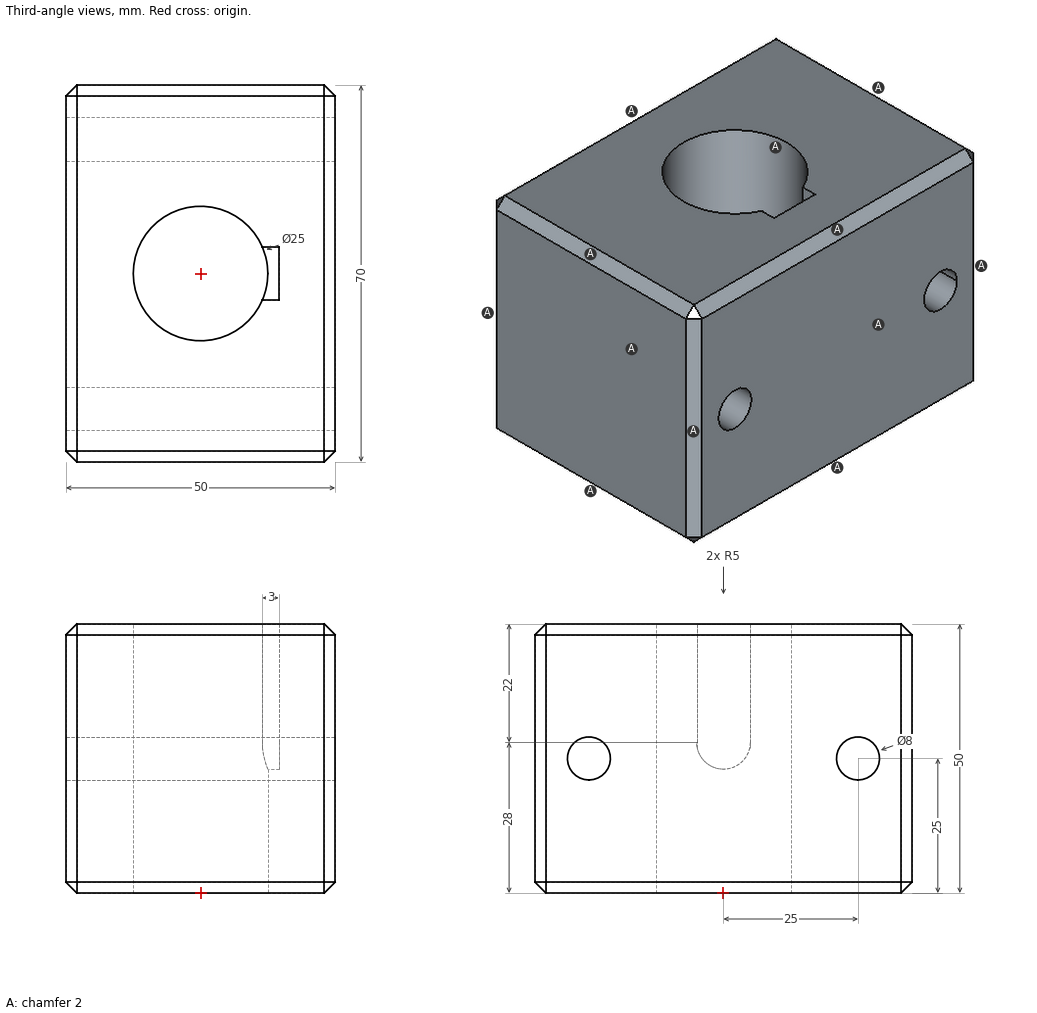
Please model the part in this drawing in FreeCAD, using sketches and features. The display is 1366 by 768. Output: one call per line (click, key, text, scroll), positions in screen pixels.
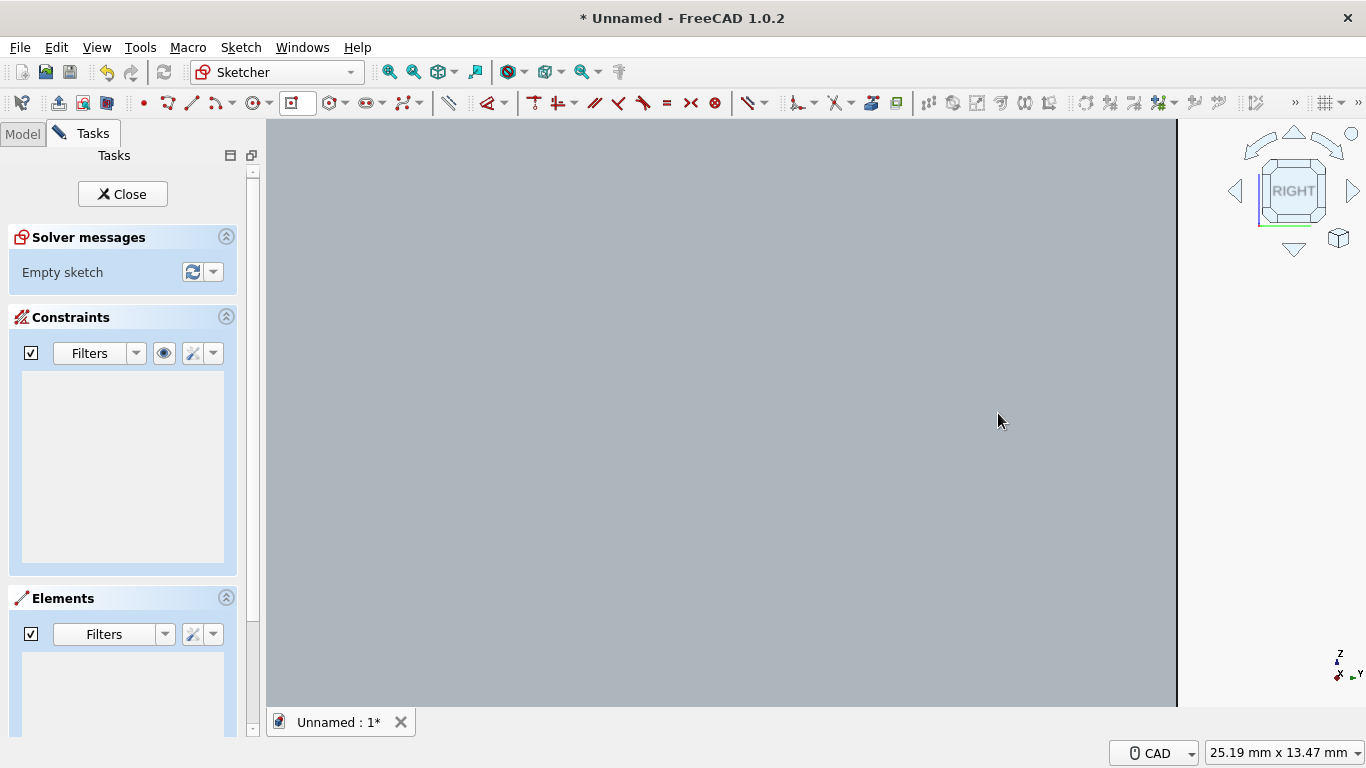
click(254, 104)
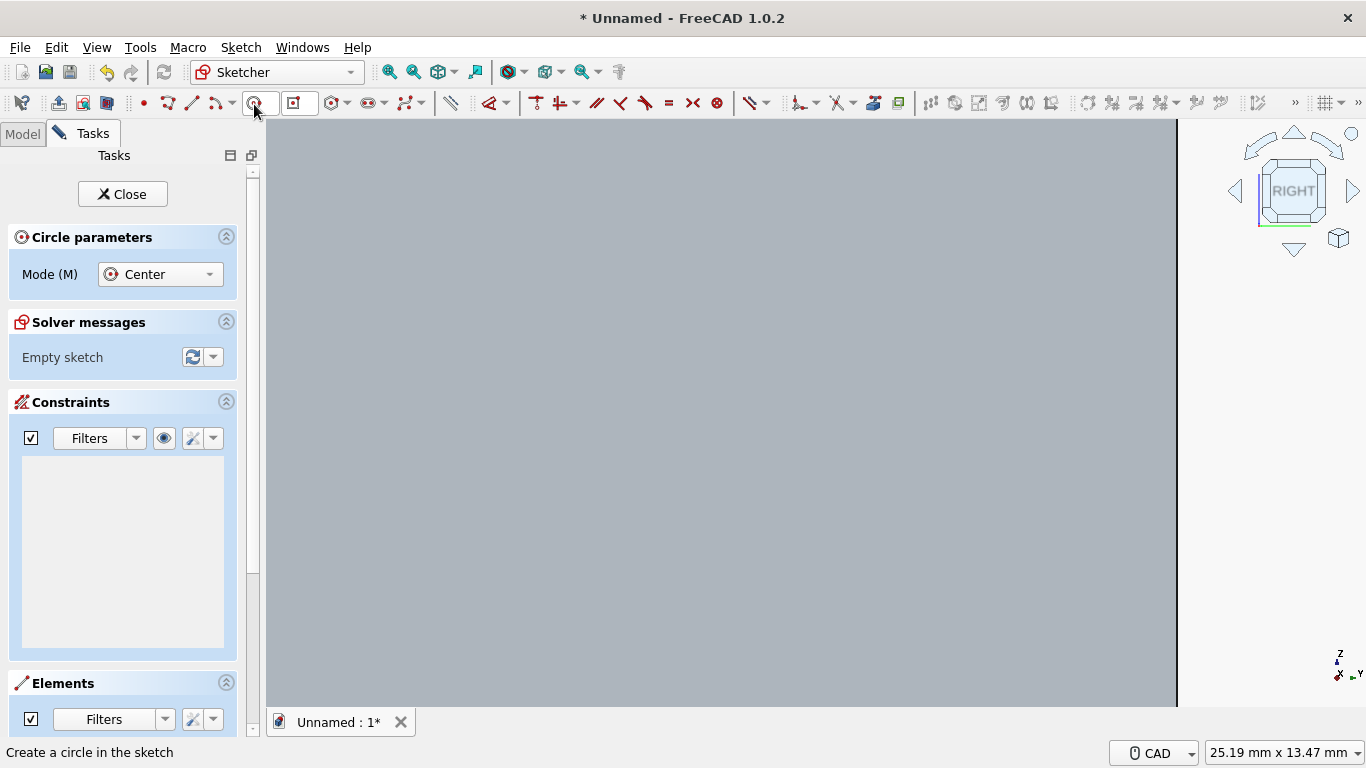
click(741, 410)
move(864, 286)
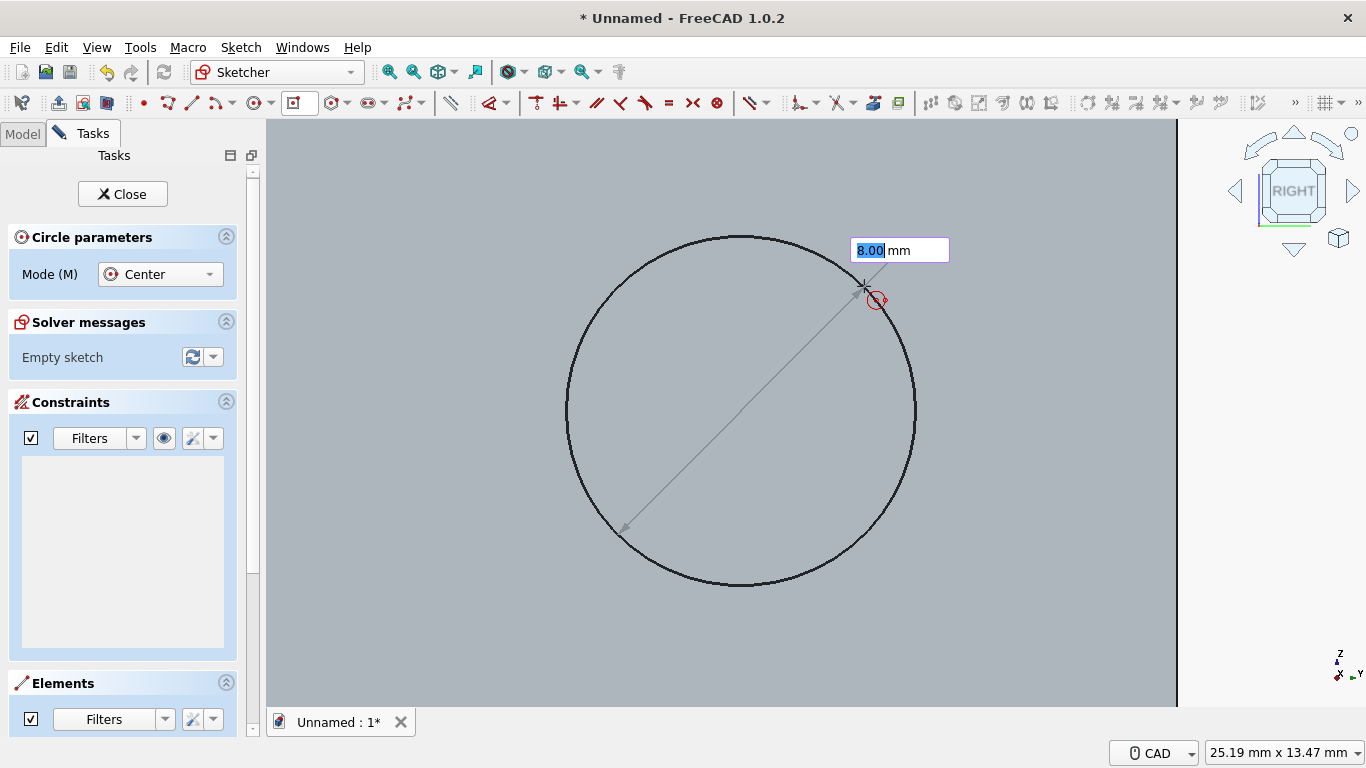
text(8)
key(Return)
key(Escape)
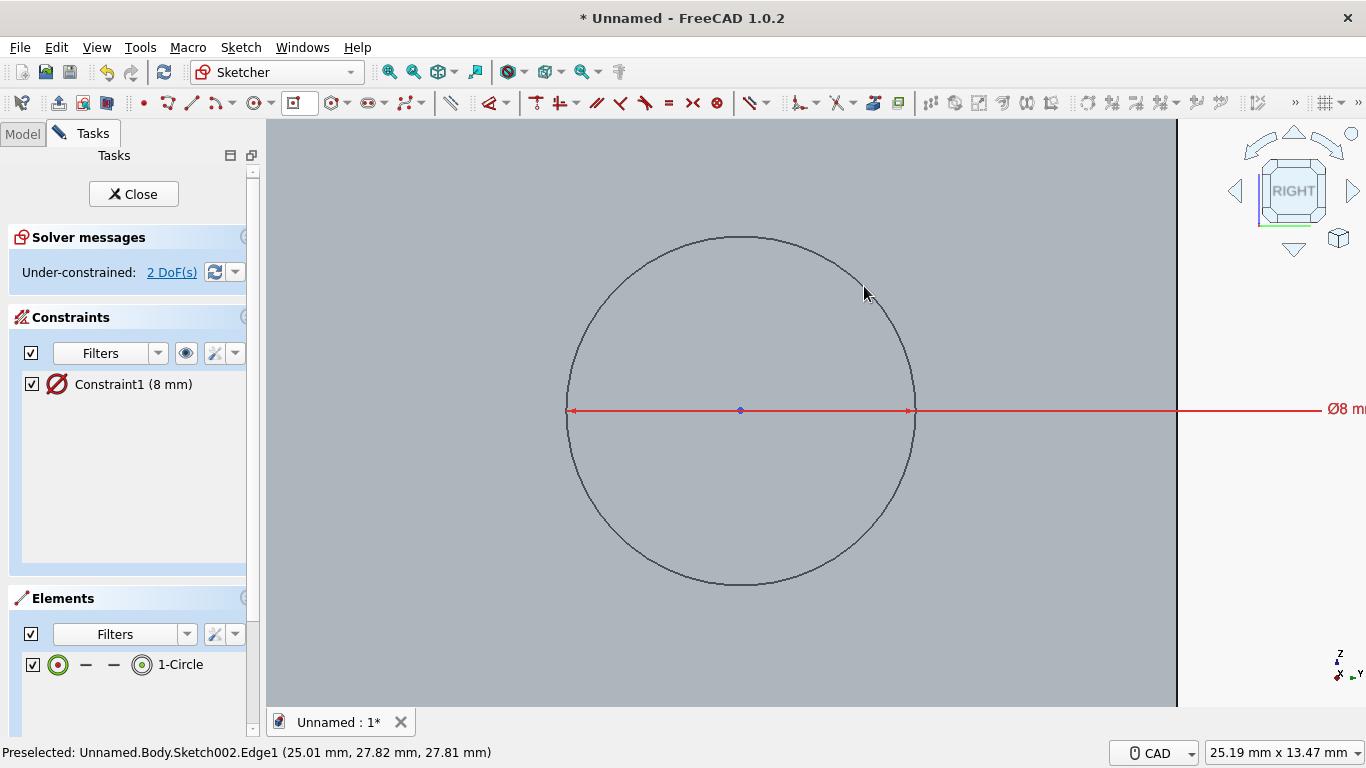
click(741, 411)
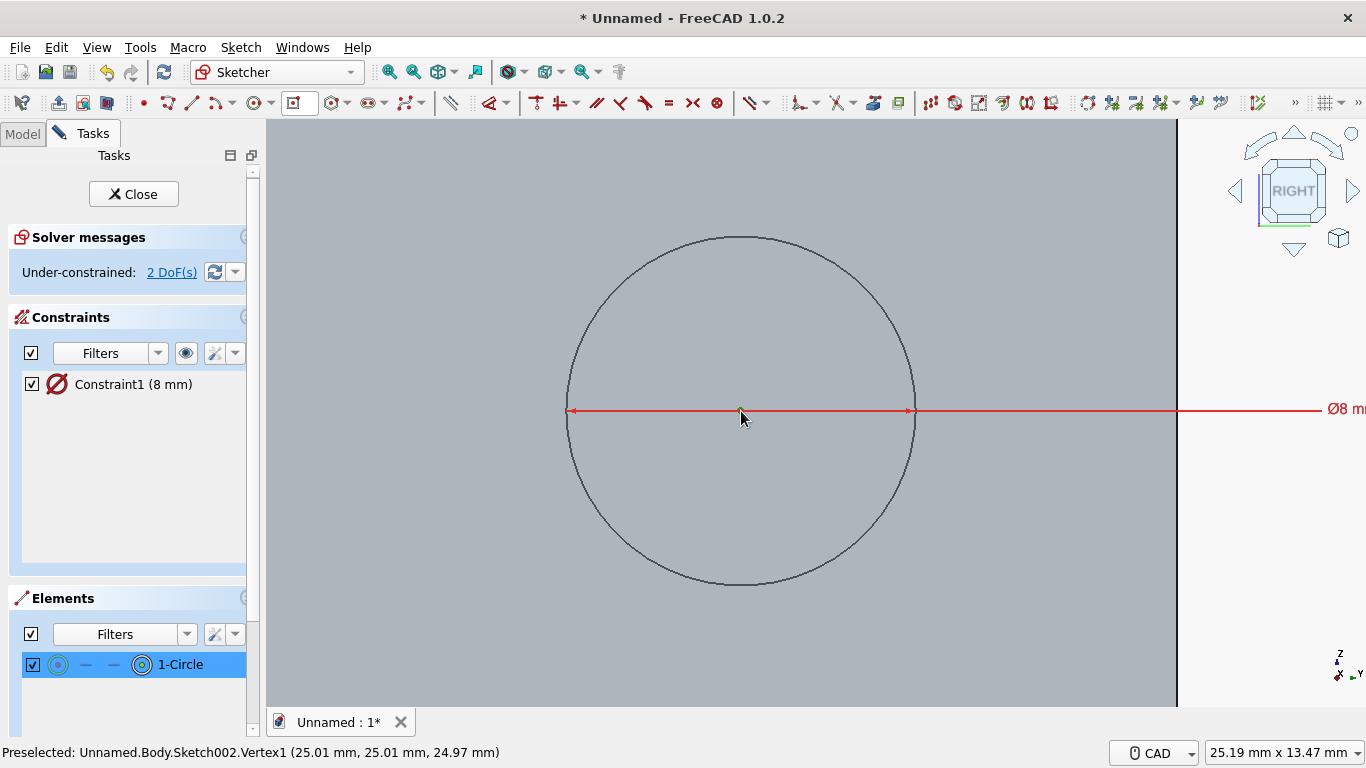
key(l)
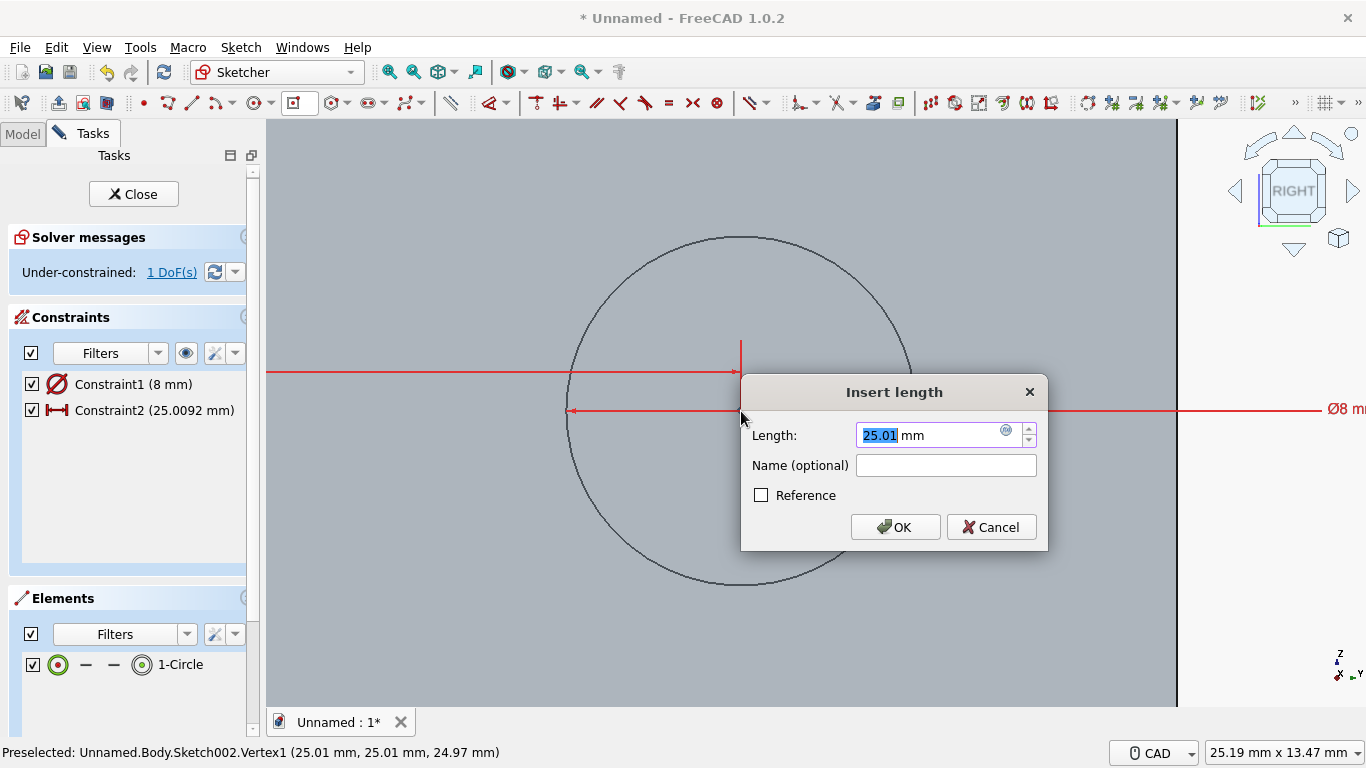
text(25)
key(Return)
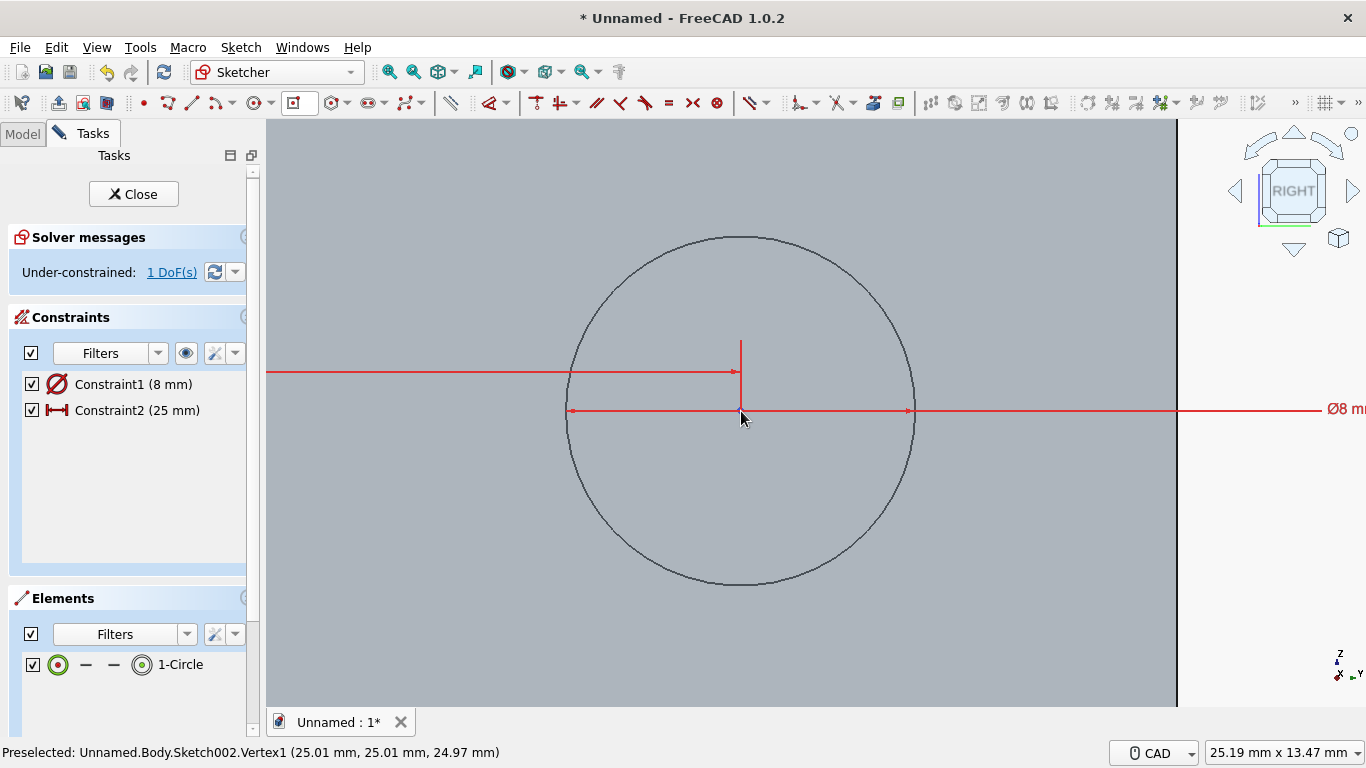
click(741, 411)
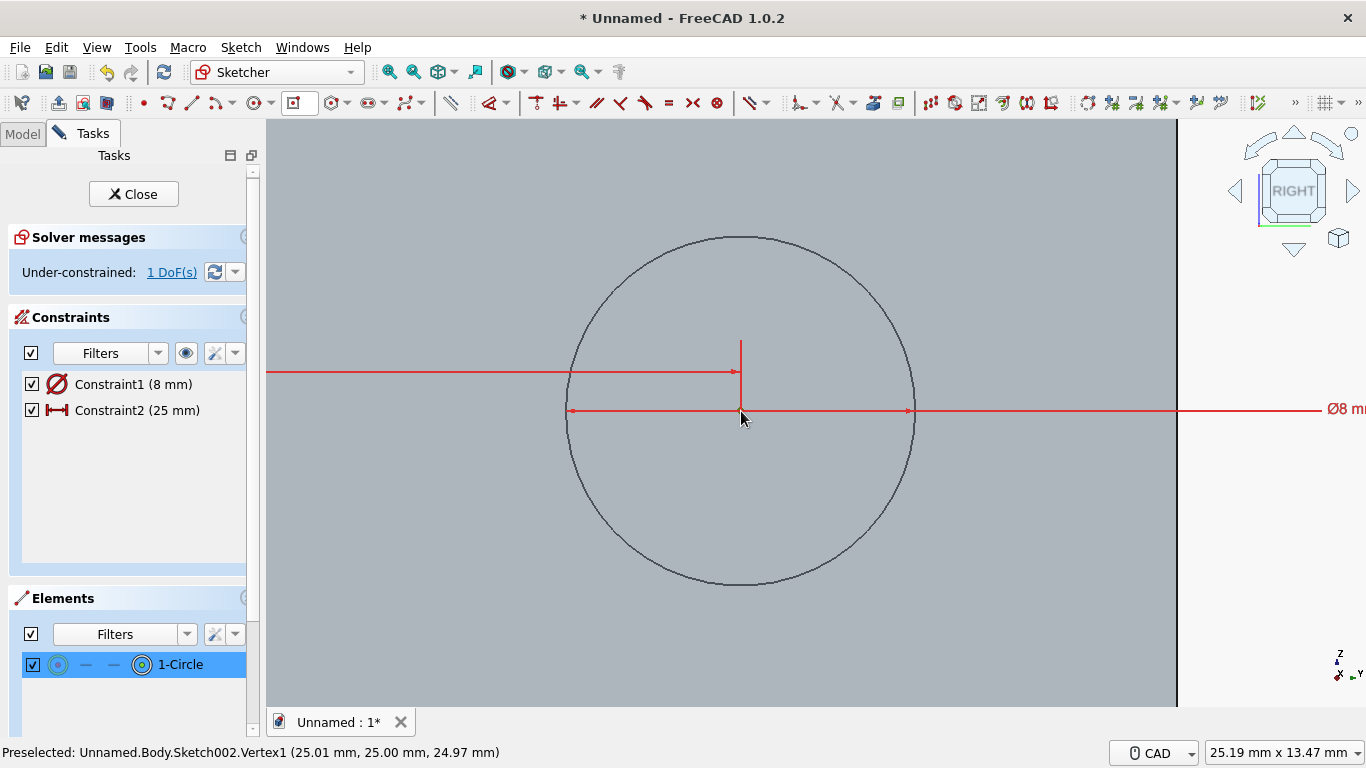
click(508, 104)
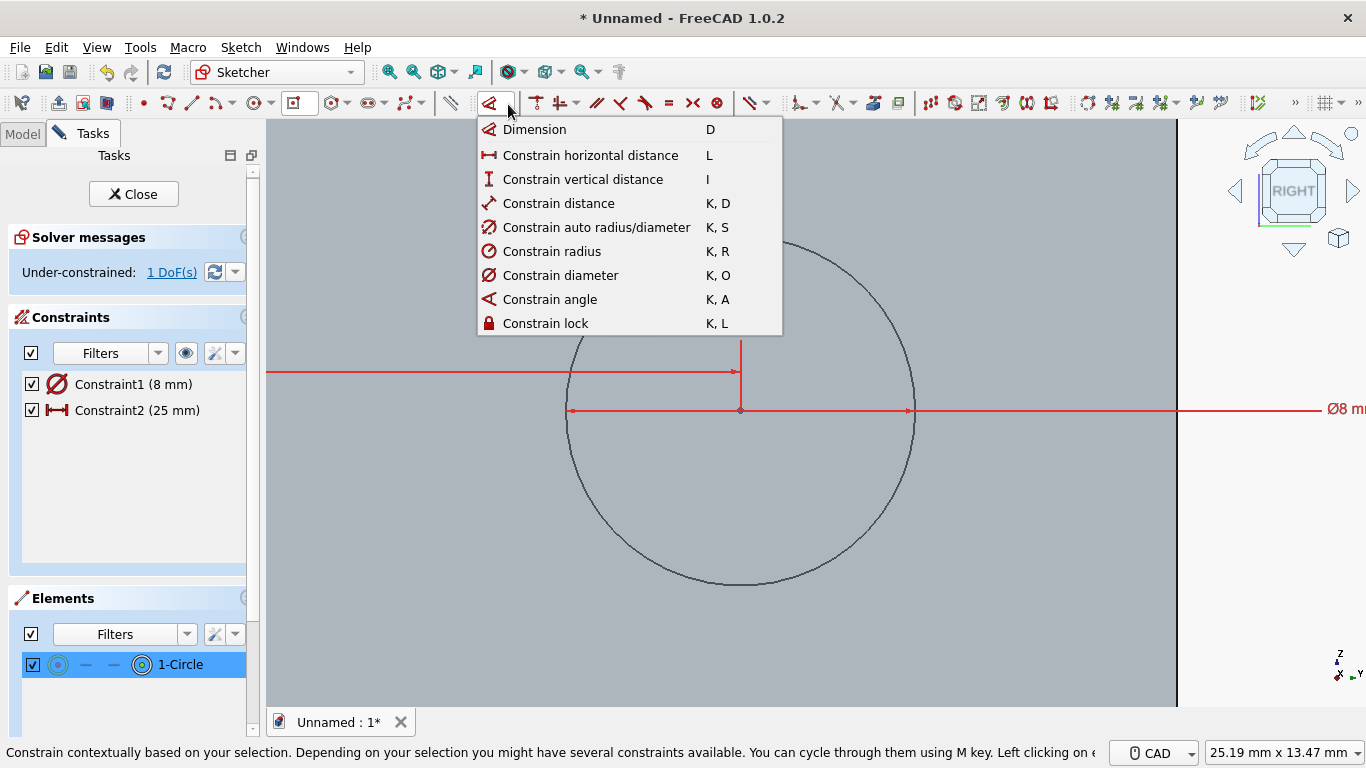
click(630, 179)